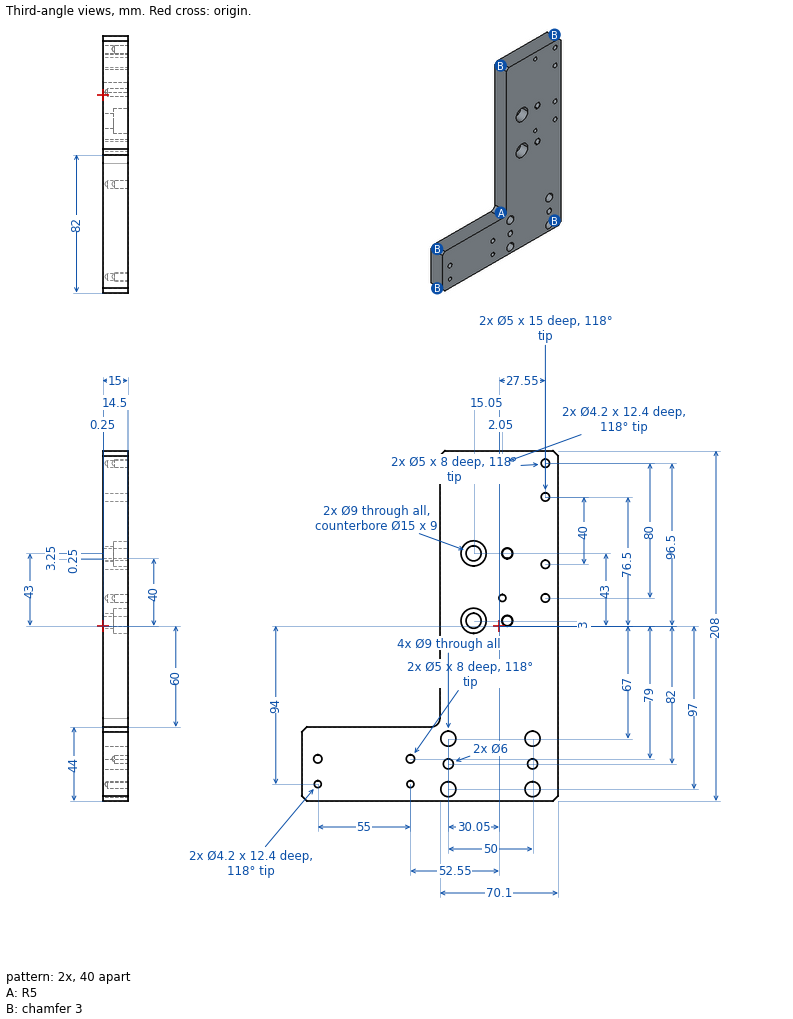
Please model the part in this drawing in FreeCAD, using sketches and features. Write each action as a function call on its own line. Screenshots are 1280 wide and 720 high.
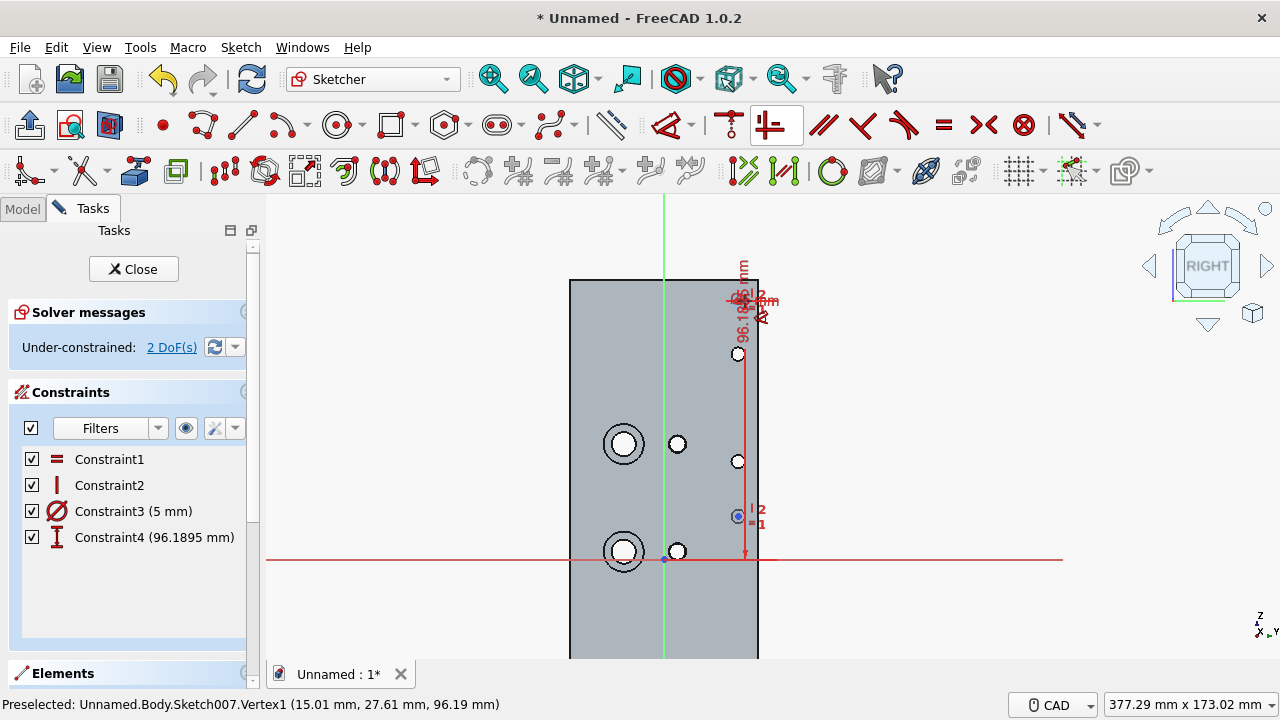
click(738, 516)
click(772, 409)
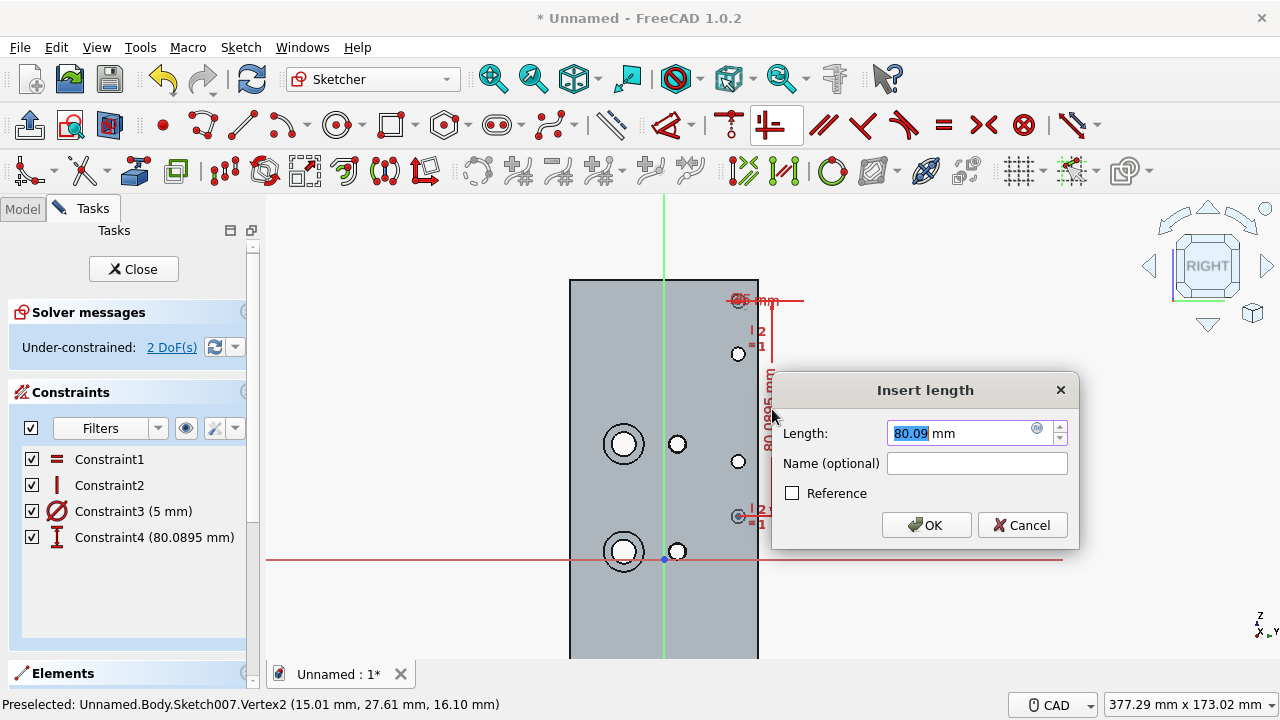
text(80)
key(Return)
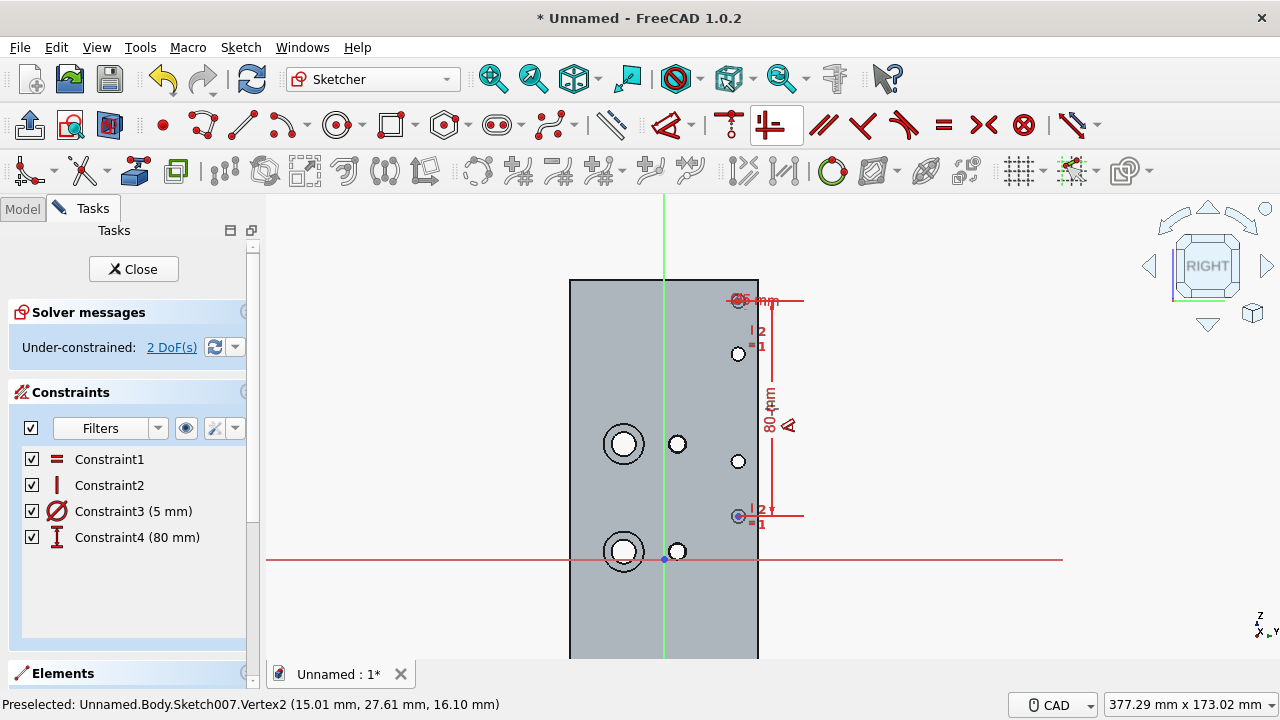
click(738, 301)
click(630, 430)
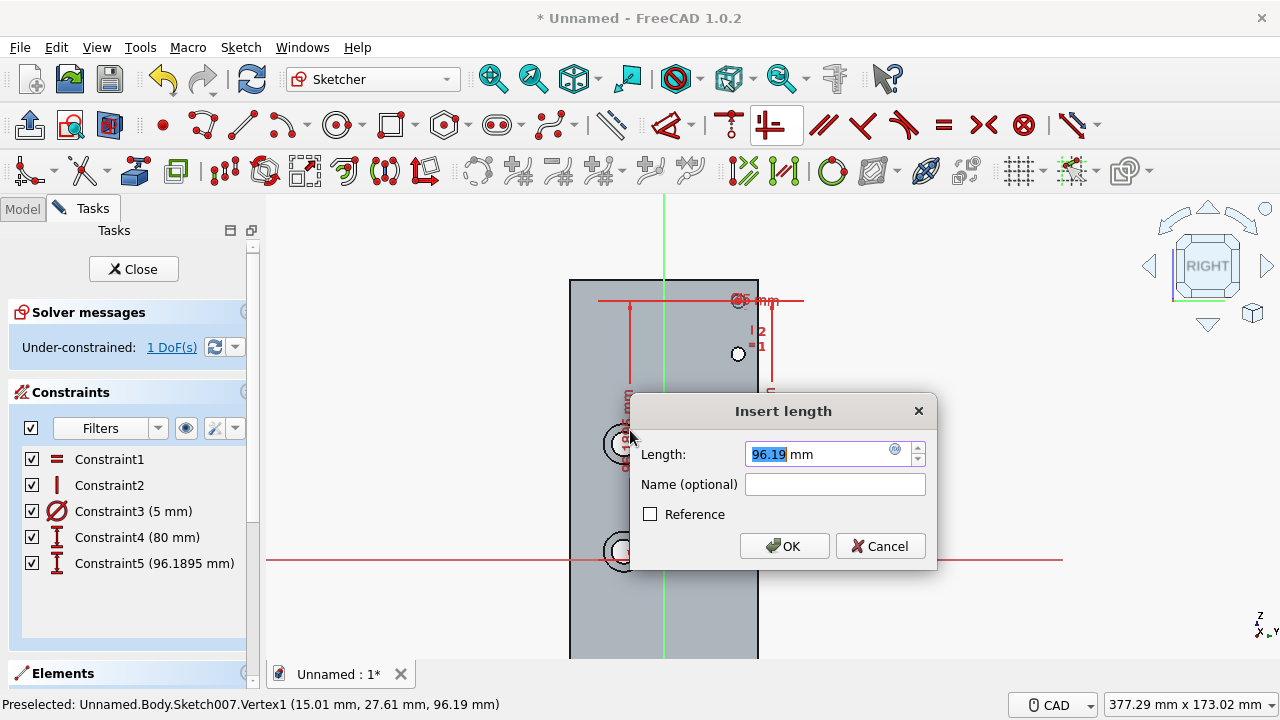
text(96.5)
key(Return)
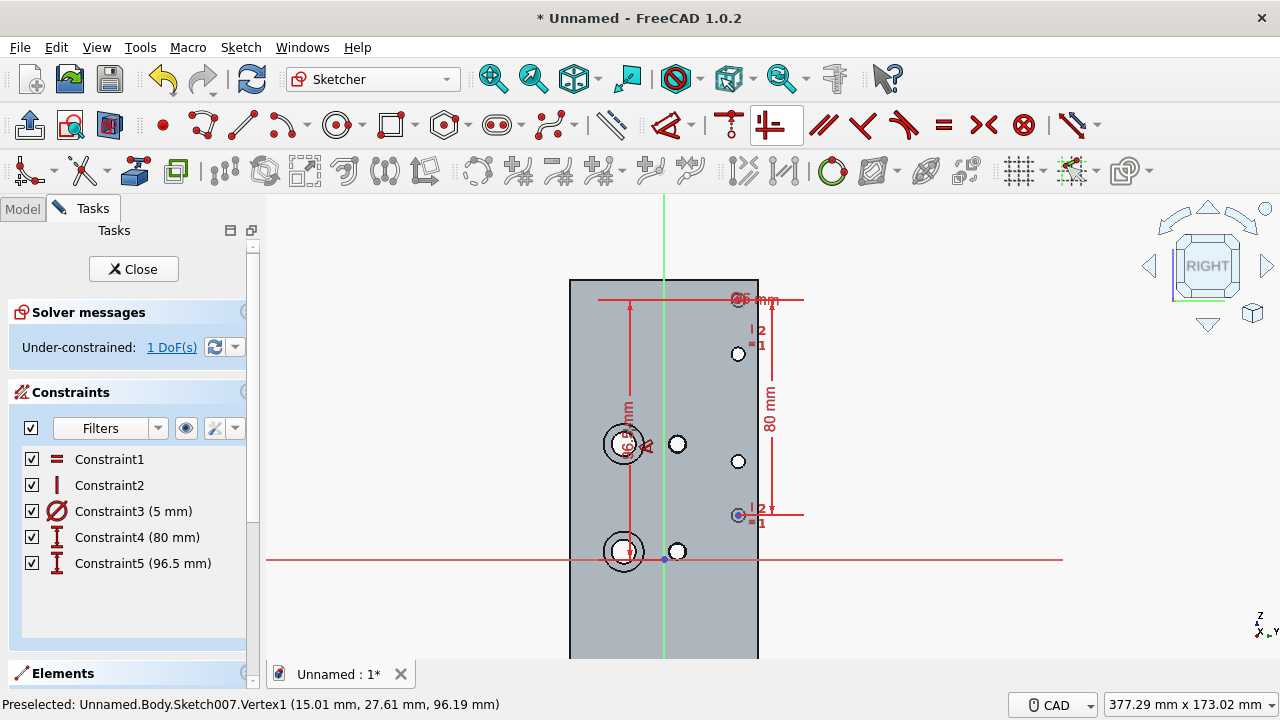
click(738, 300)
click(701, 594)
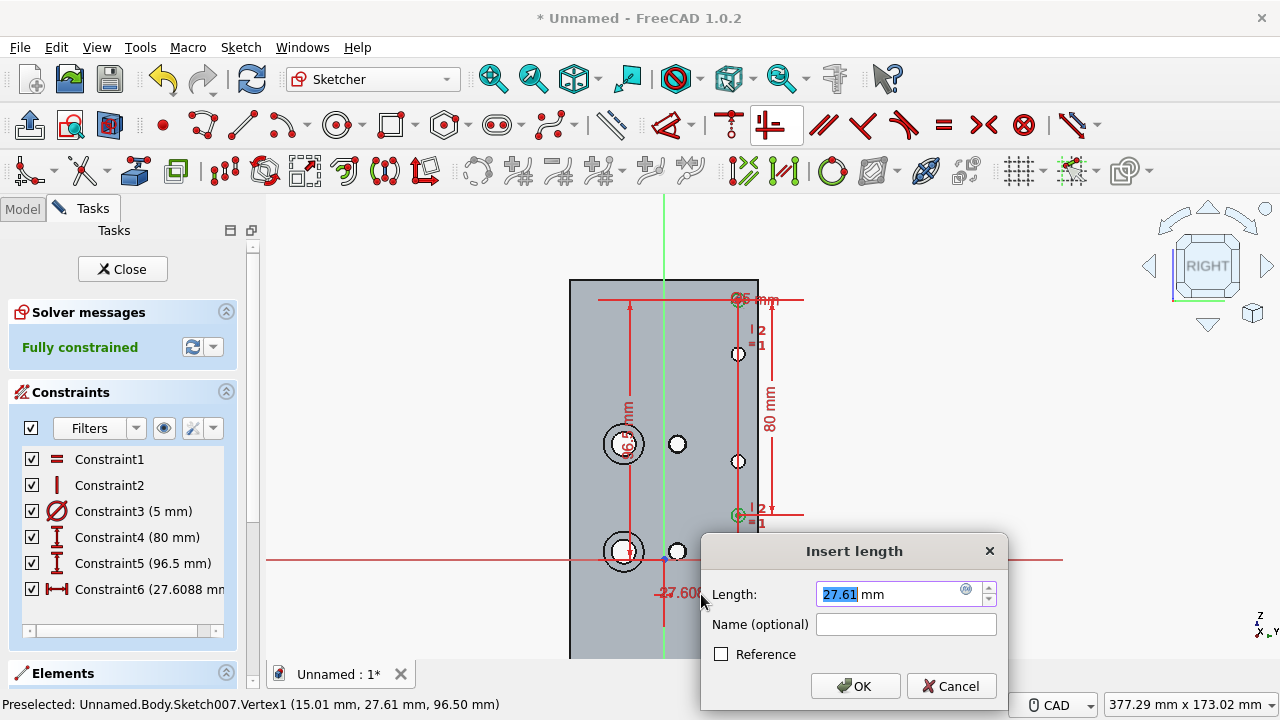
text(27.55)
key(Return)
key(Escape)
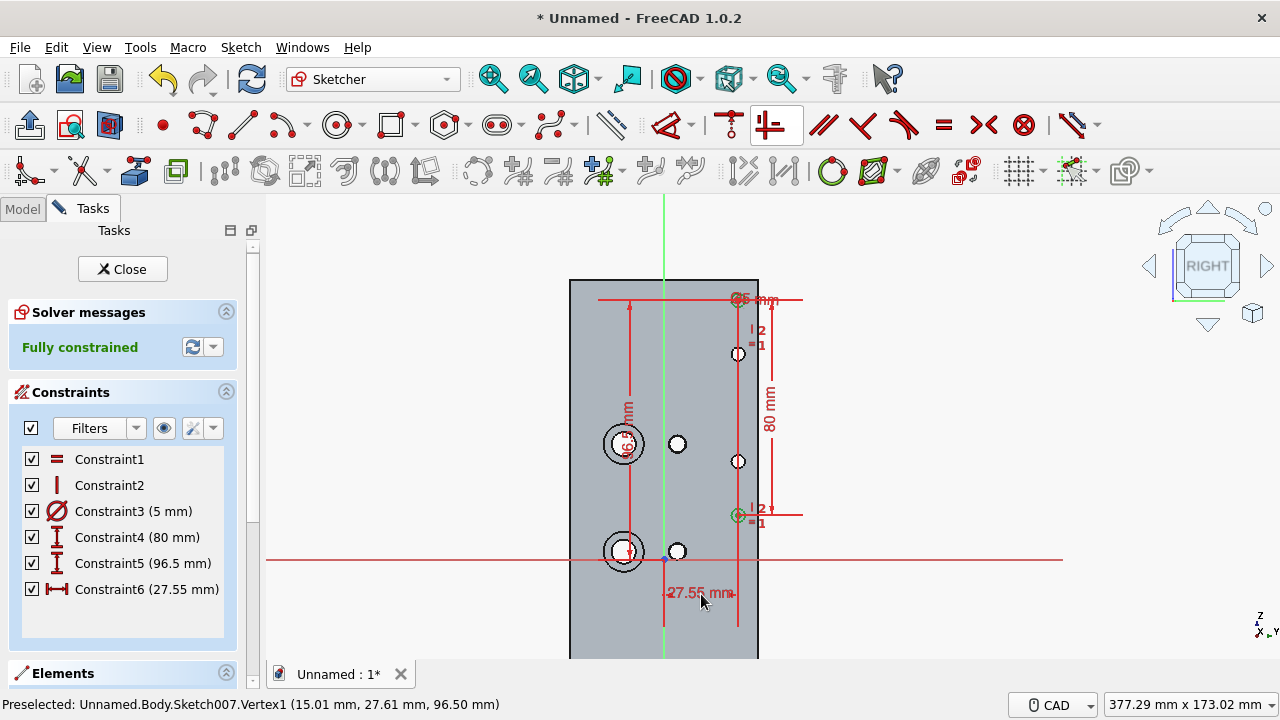
click(123, 269)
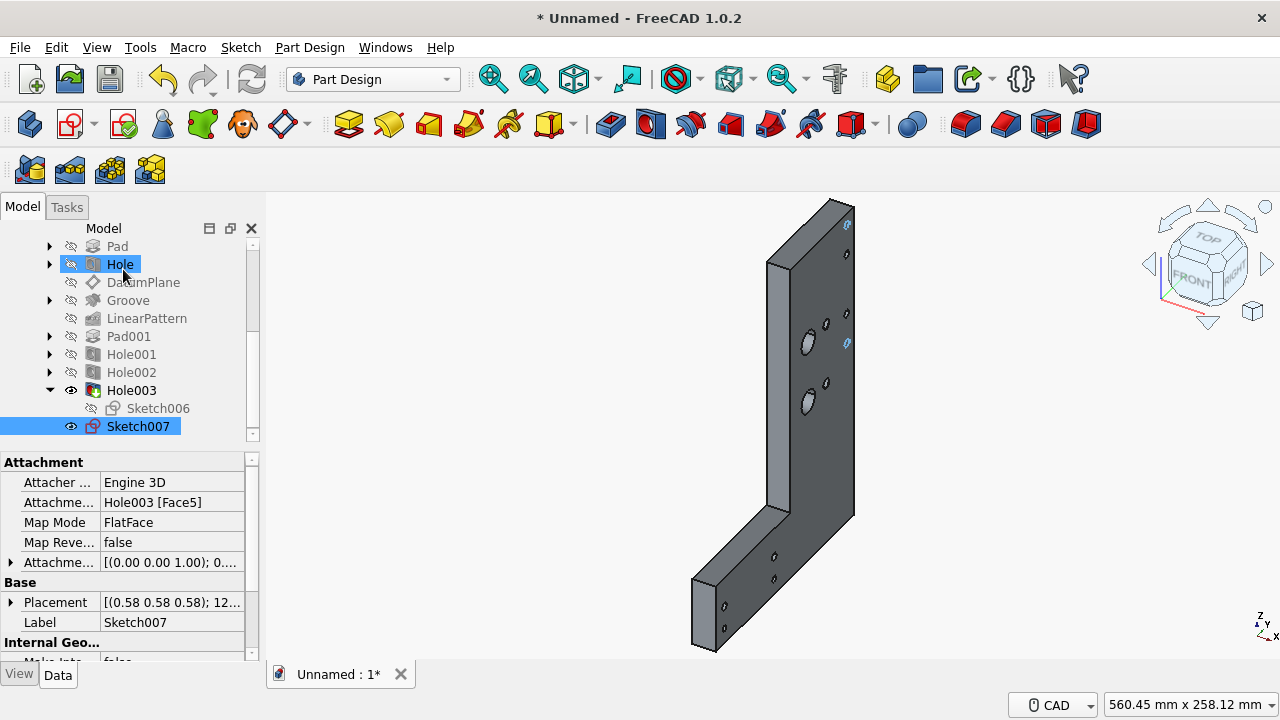
click(652, 124)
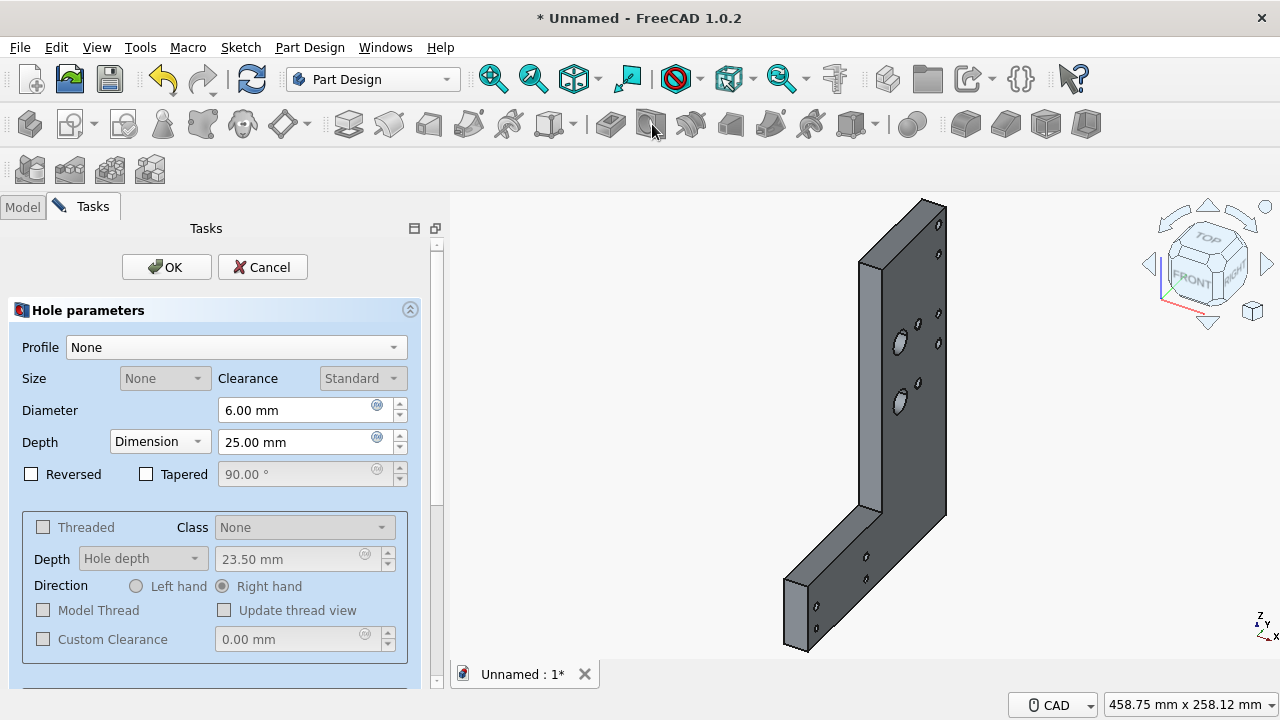
triple_click(305, 410)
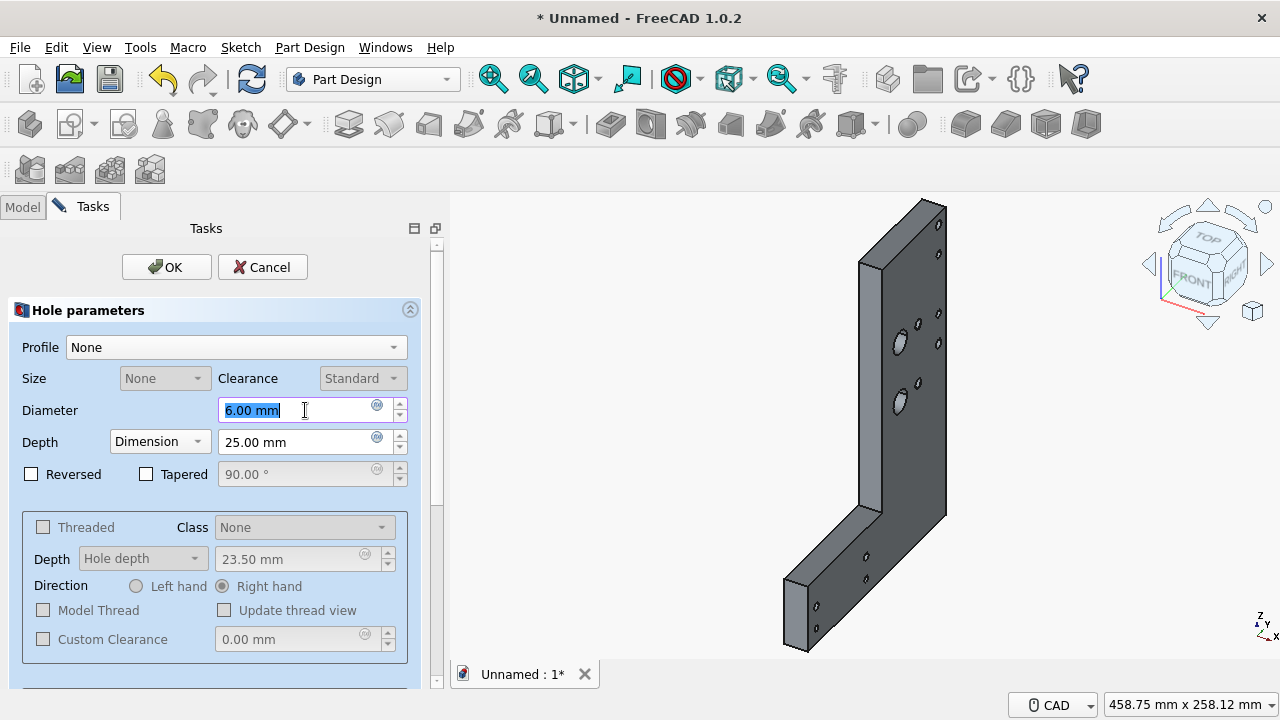
text(5)
key(Tab)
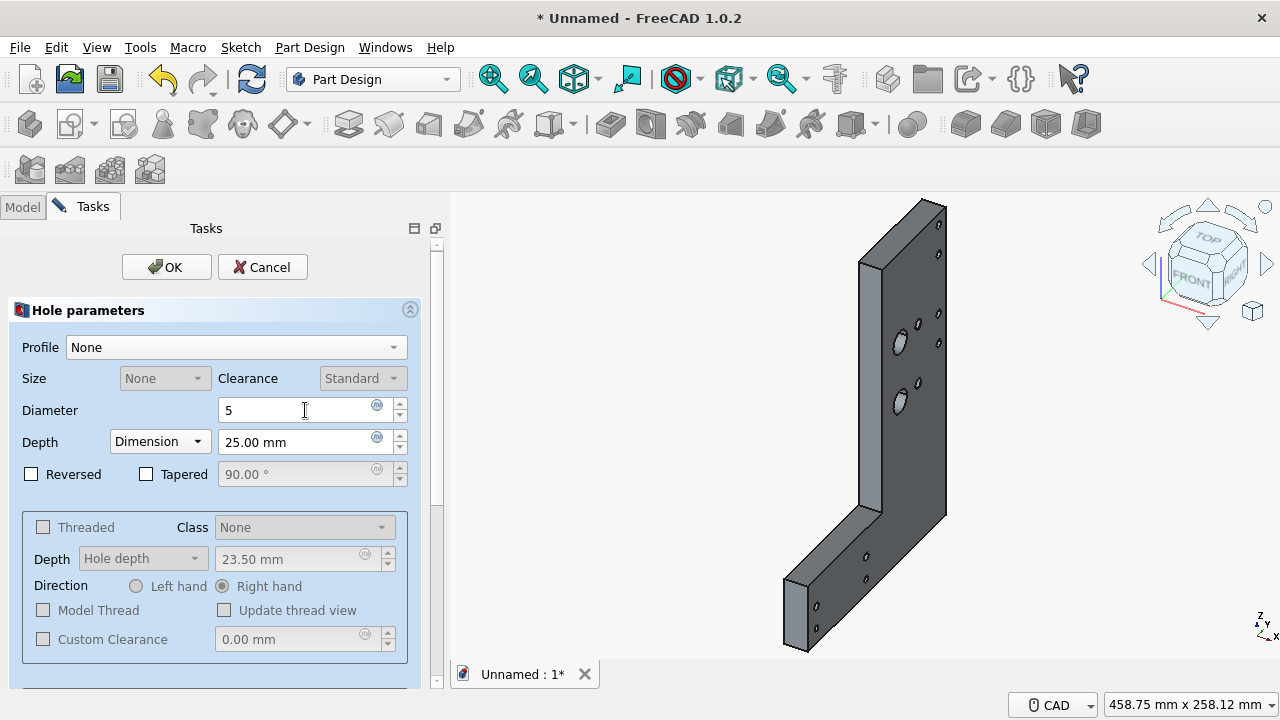
triple_click(305, 442)